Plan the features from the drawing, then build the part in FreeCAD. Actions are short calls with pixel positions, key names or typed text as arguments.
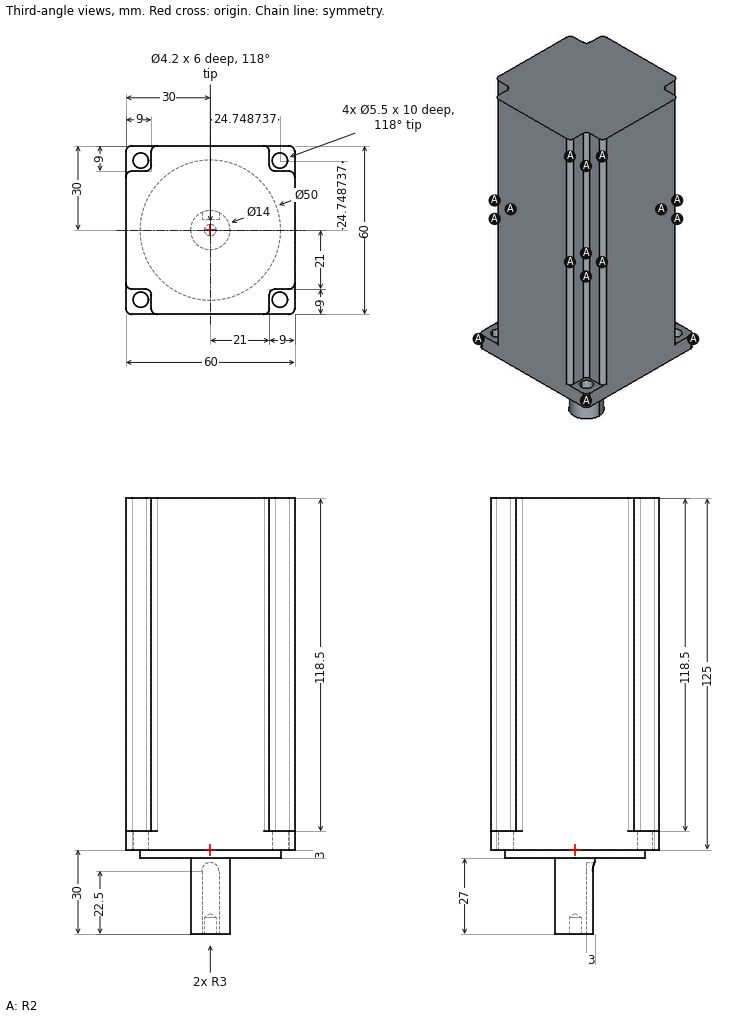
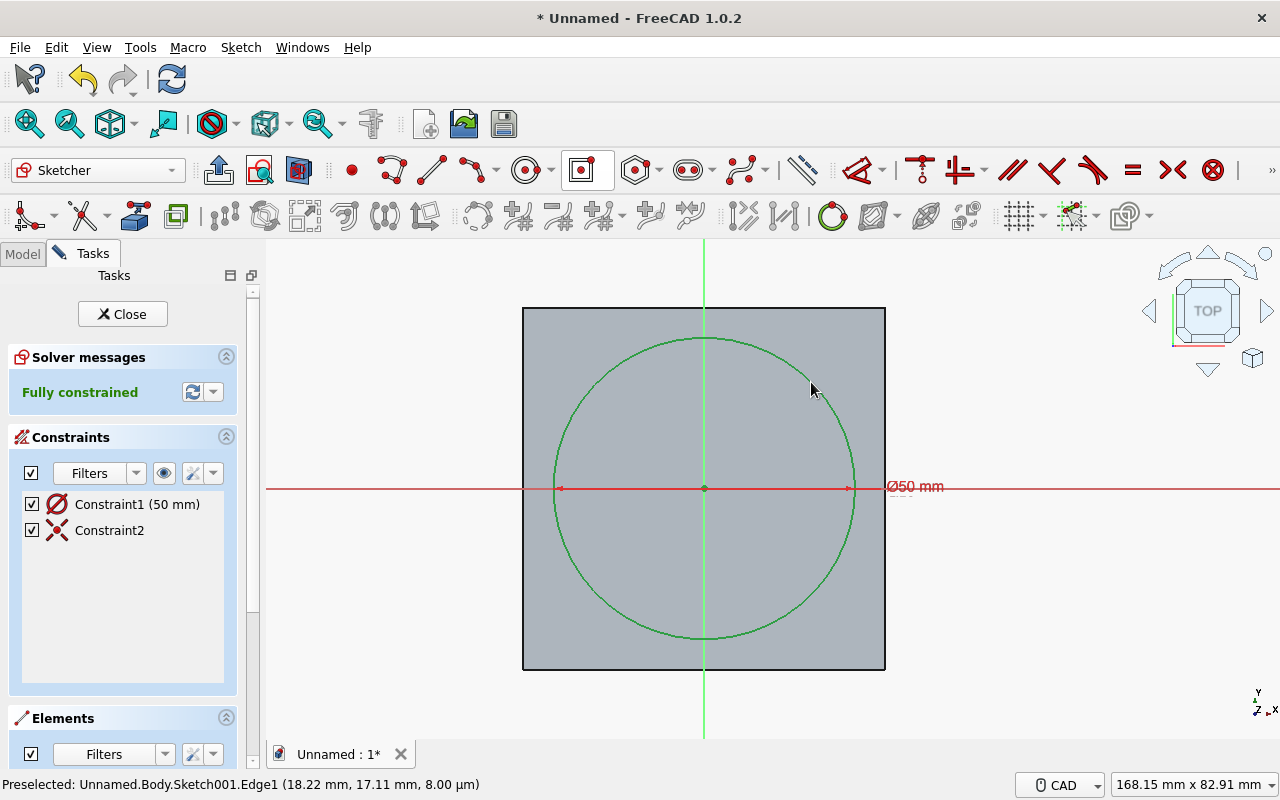
click(123, 314)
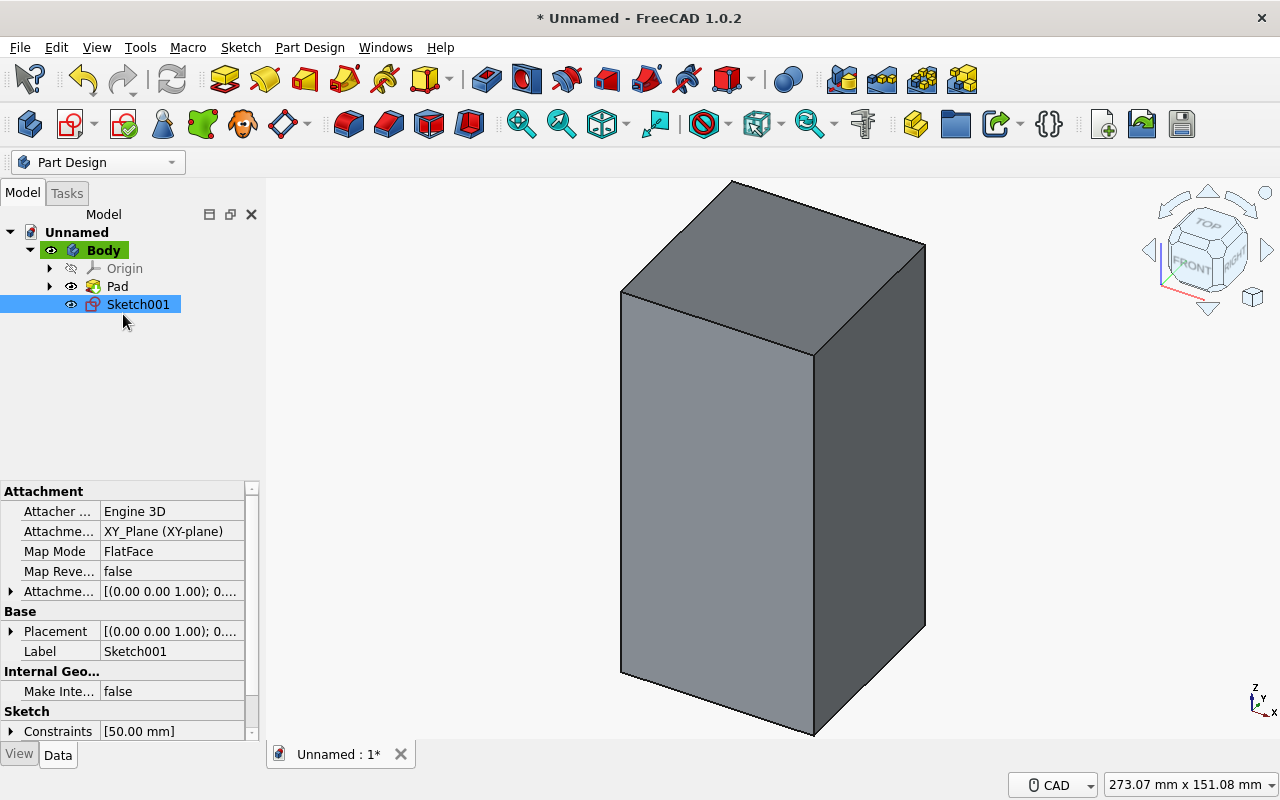
click(226, 80)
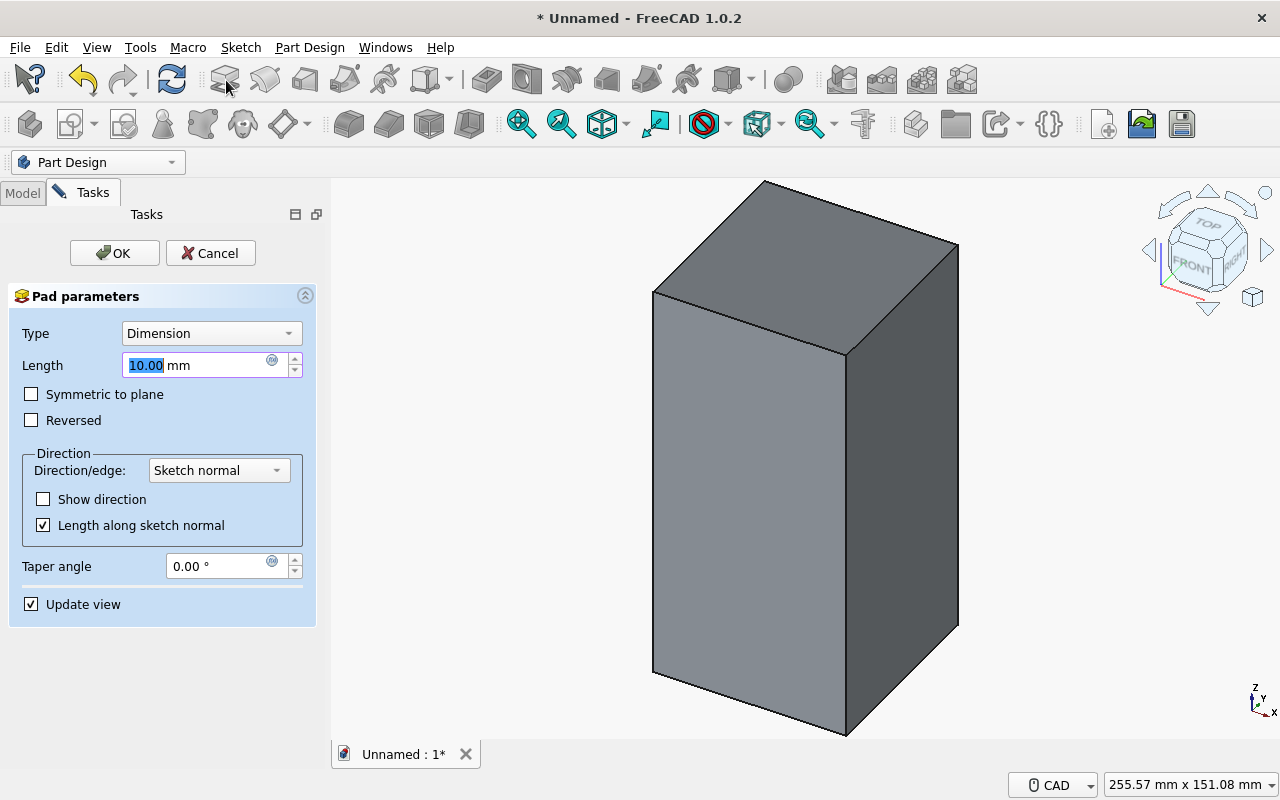
text(3)
key(Tab)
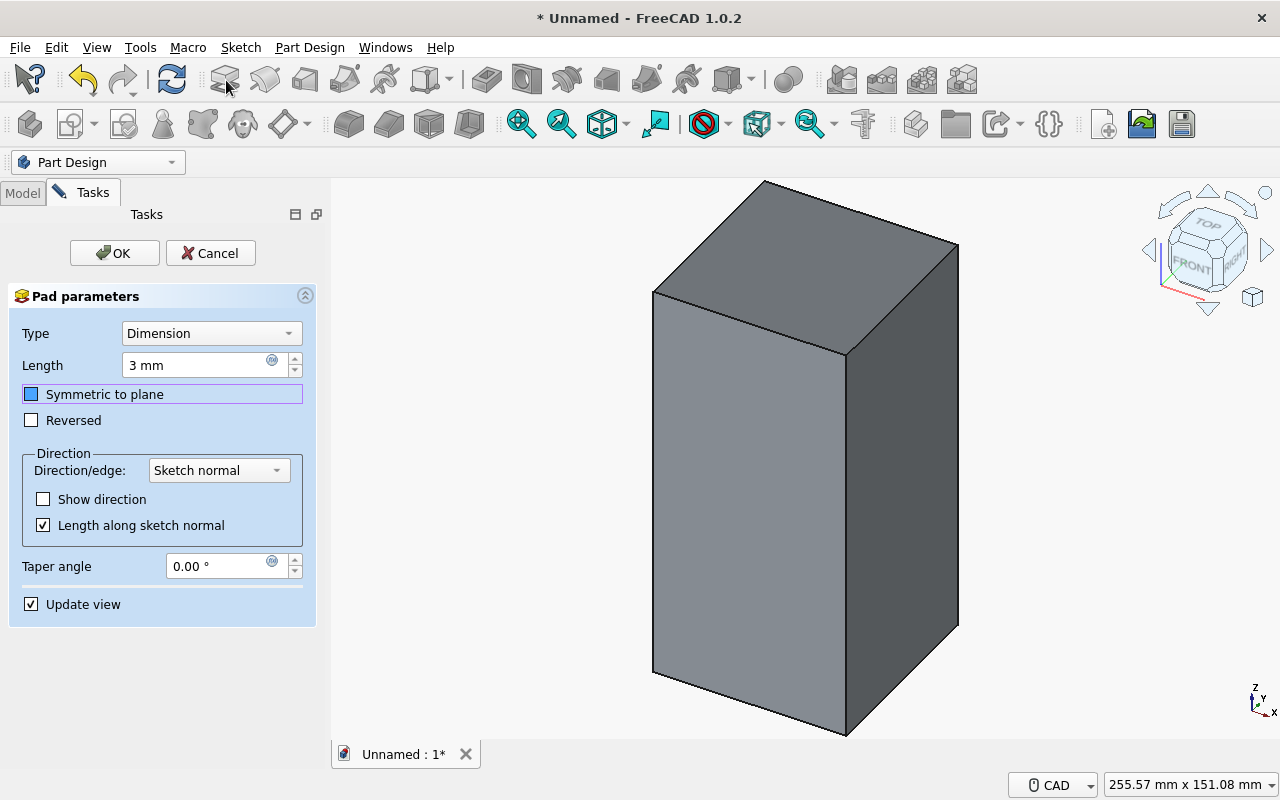
click(30, 420)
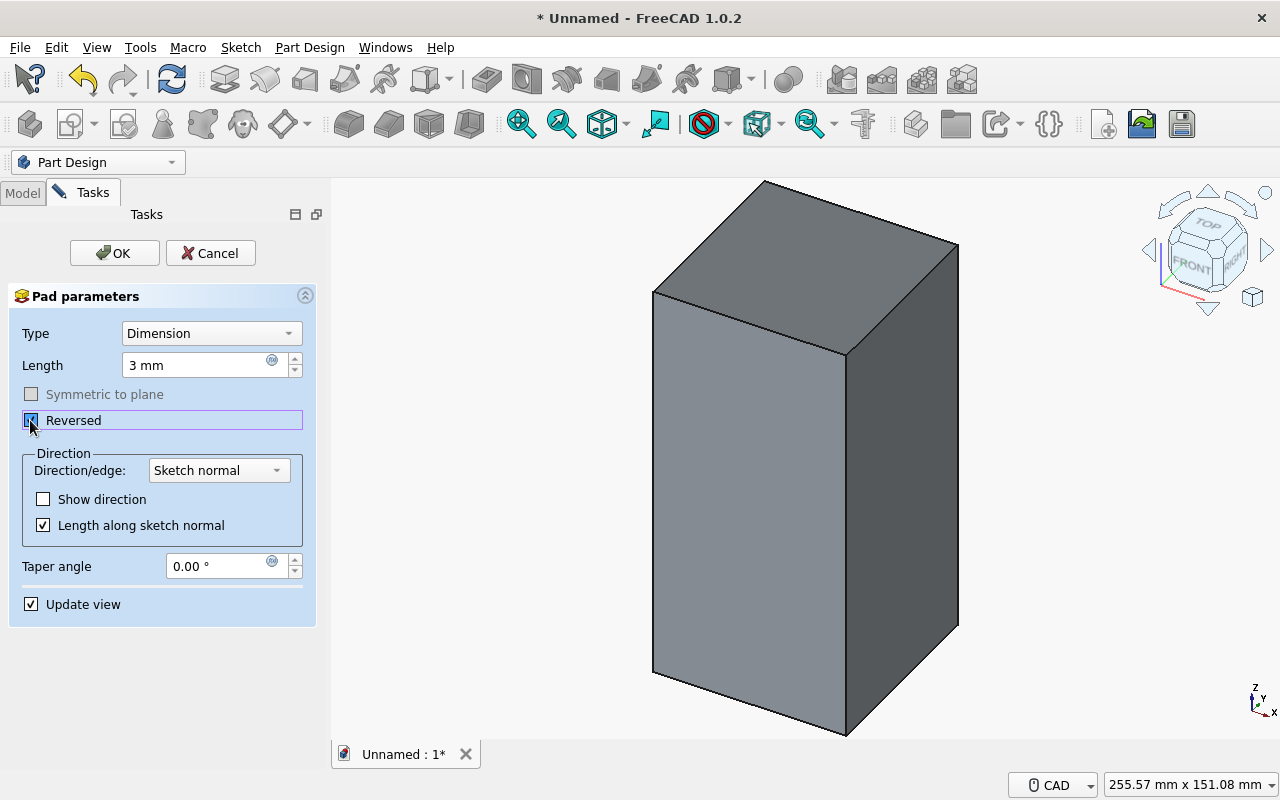
click(115, 253)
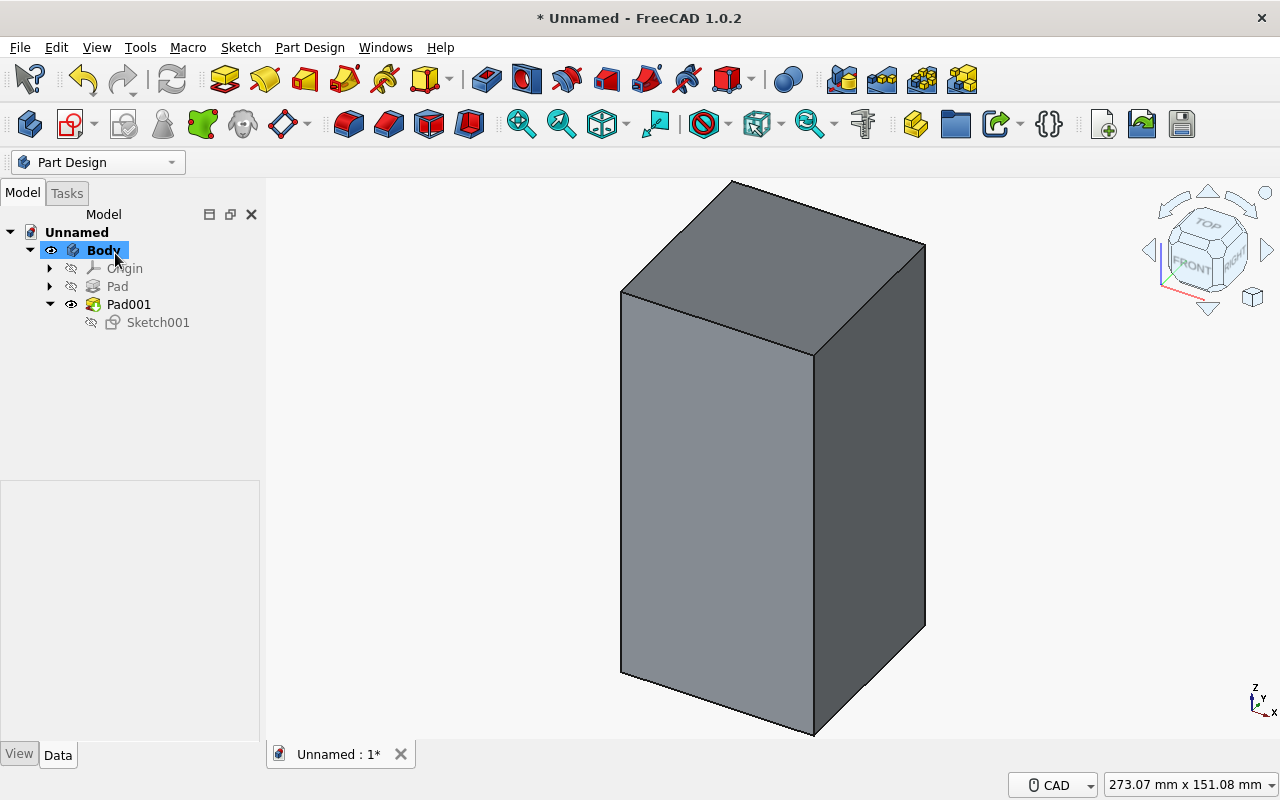
click(522, 124)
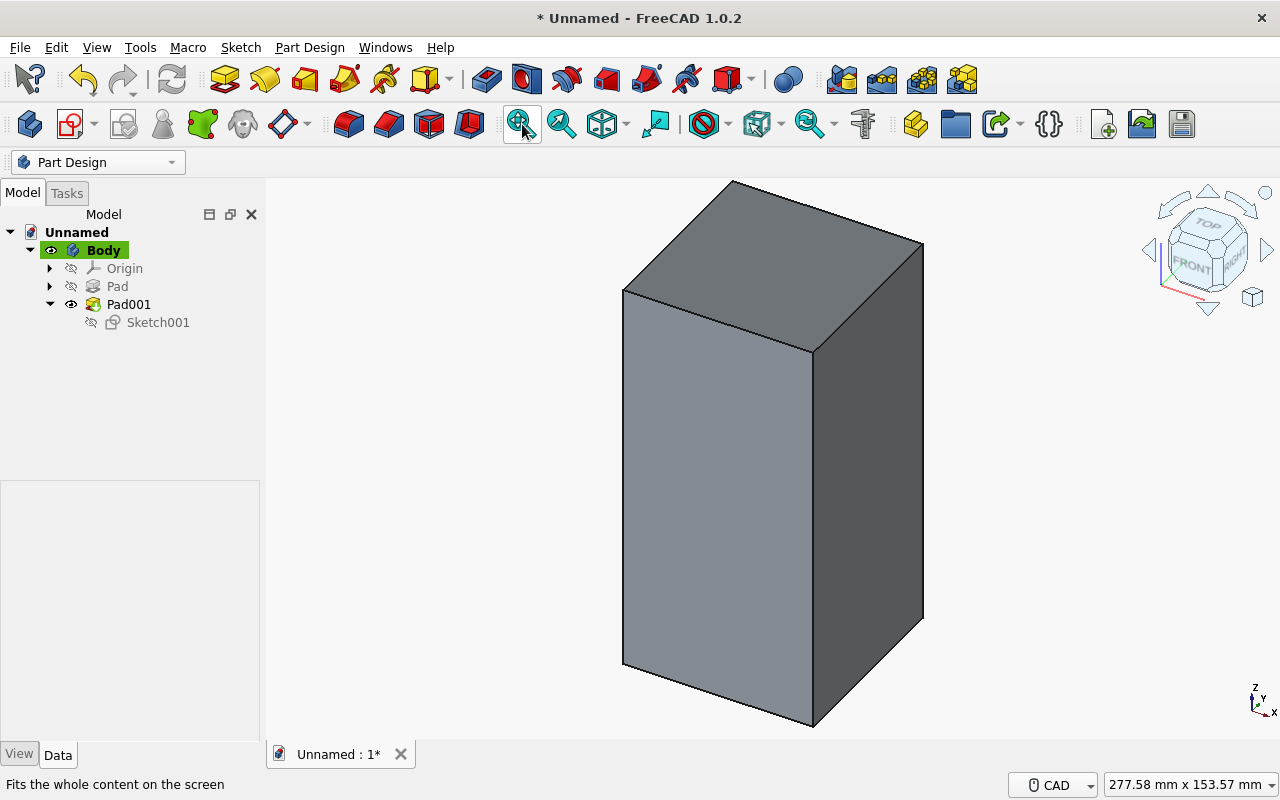
key(5)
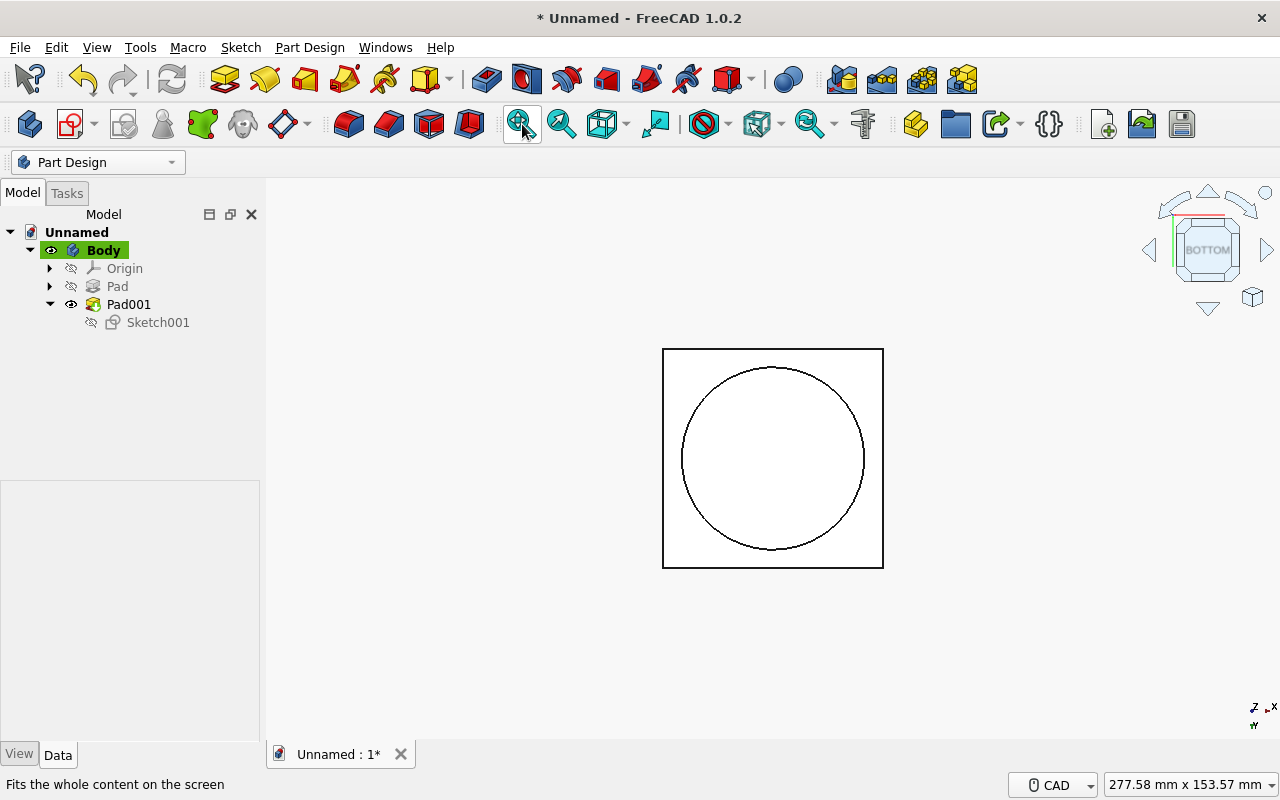
key(v)
key(f)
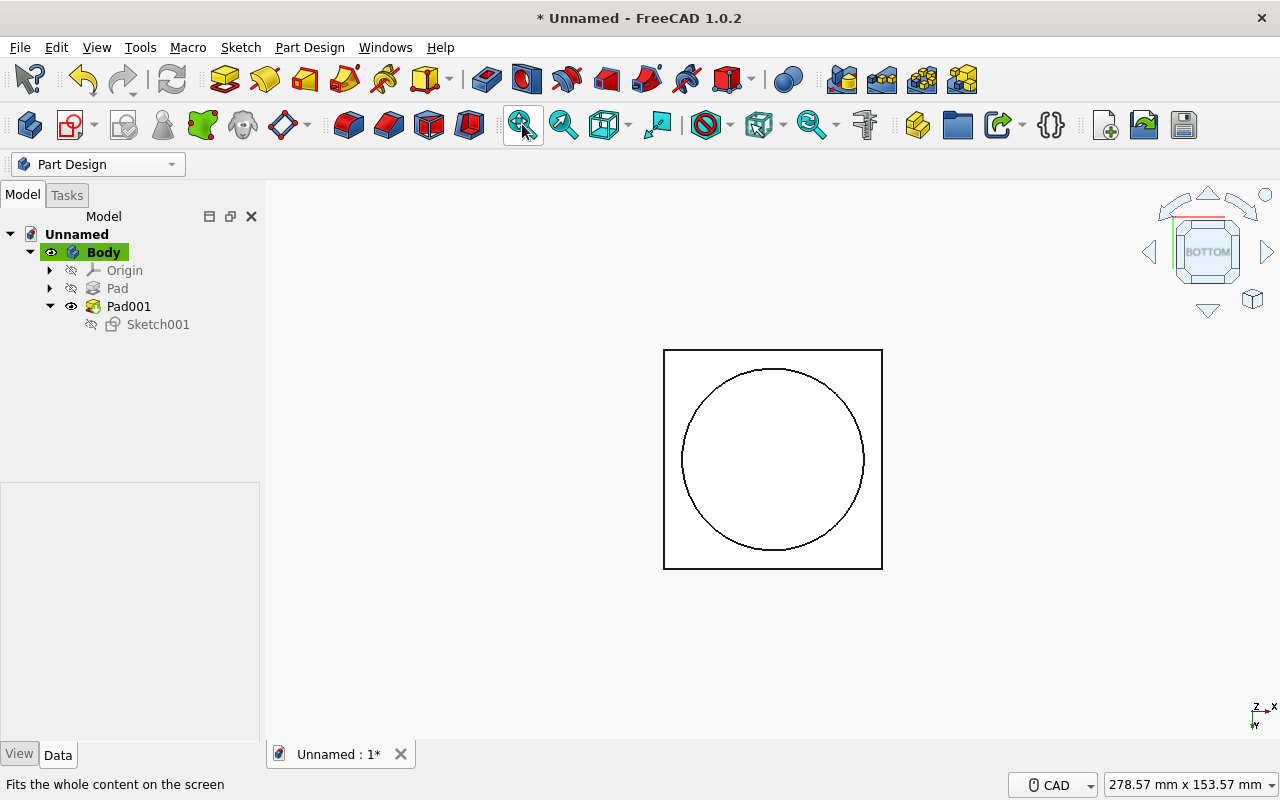
click(773, 458)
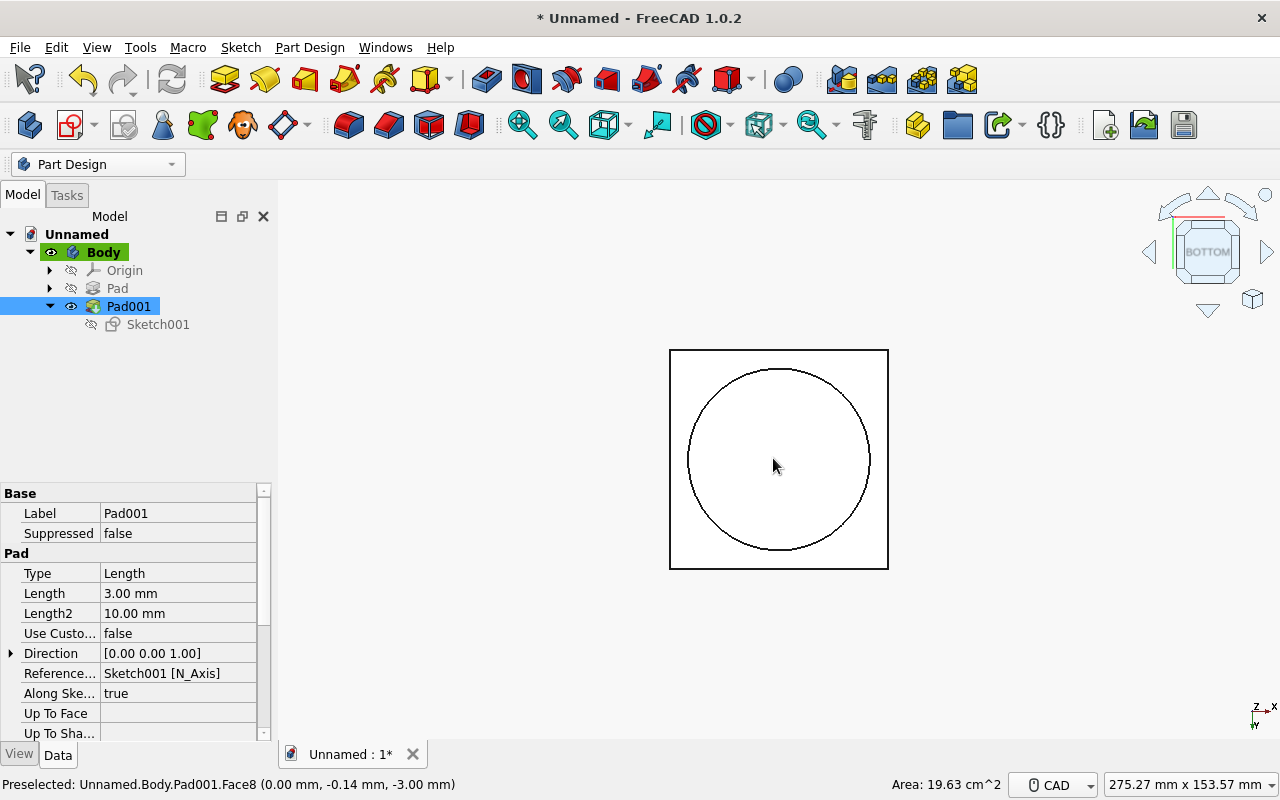
click(70, 126)